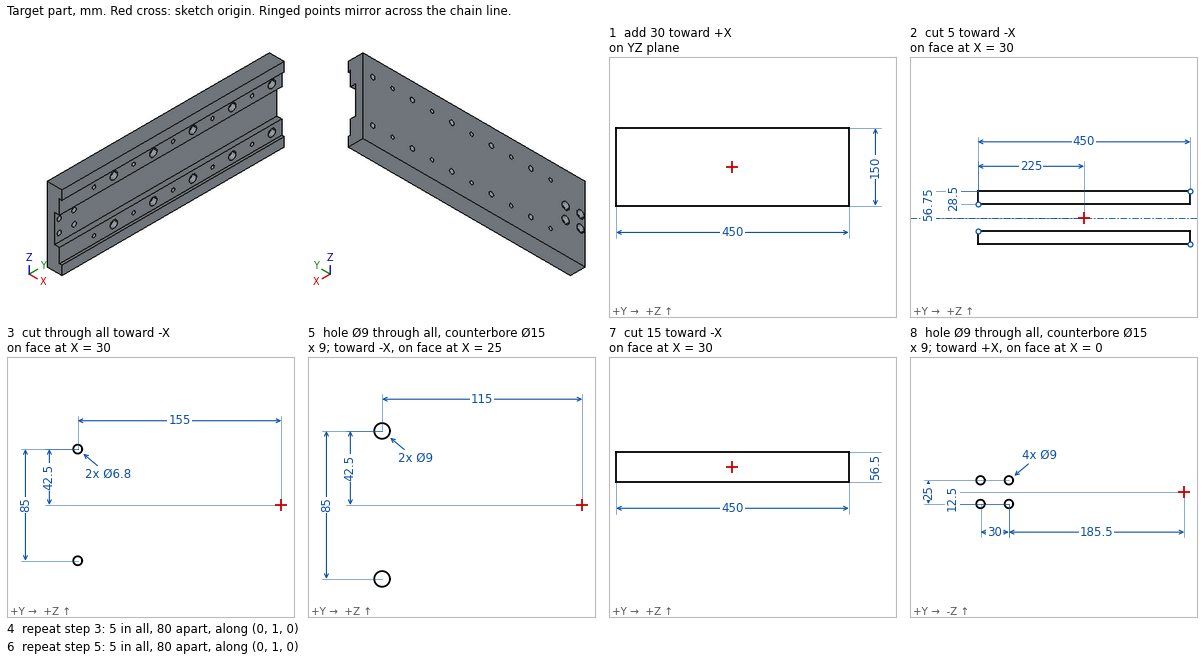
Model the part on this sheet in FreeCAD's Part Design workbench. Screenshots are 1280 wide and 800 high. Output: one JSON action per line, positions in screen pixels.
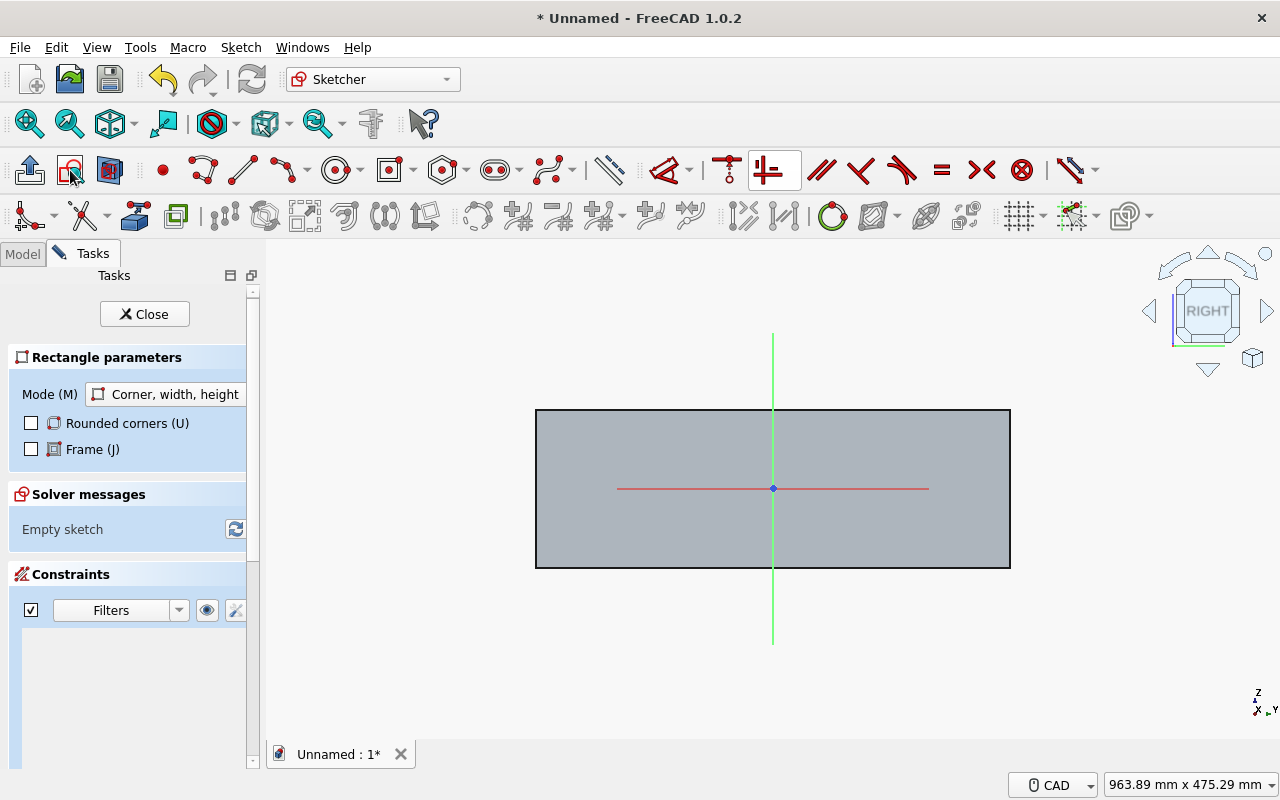
{"action": "left_click", "coordinate": [536, 429]}
{"action": "left_click", "coordinate": [1010, 459]}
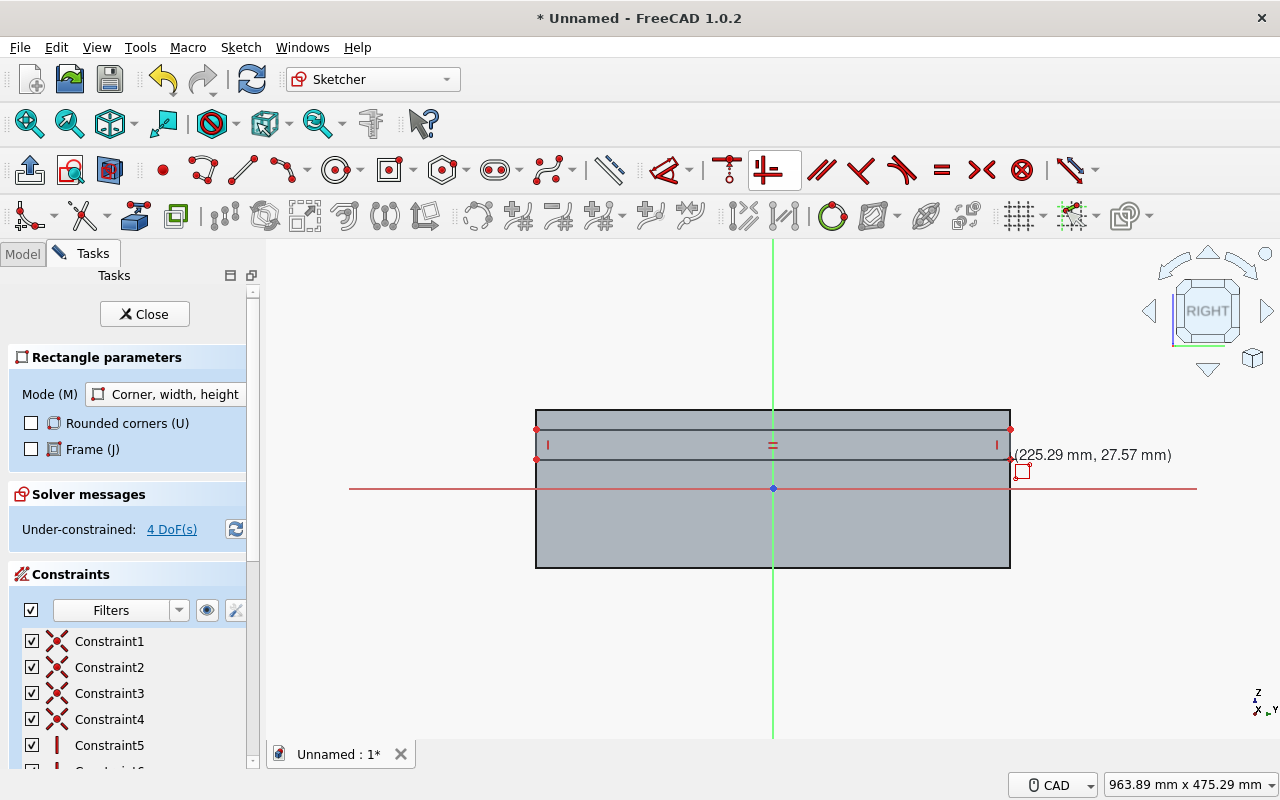
{"action": "left_click", "coordinate": [536, 519]}
{"action": "left_click", "coordinate": [1010, 549]}
{"action": "key", "text": "Escape"}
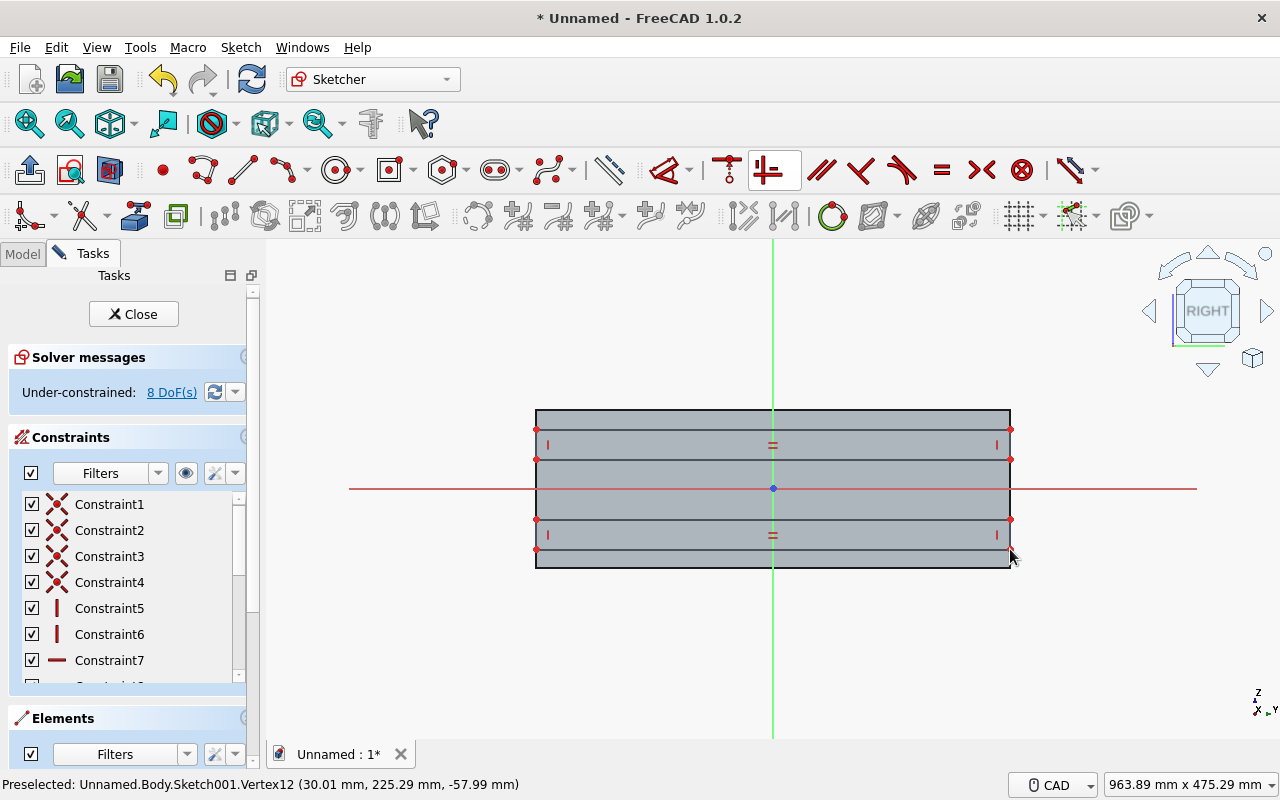
{"action": "left_click", "coordinate": [536, 460]}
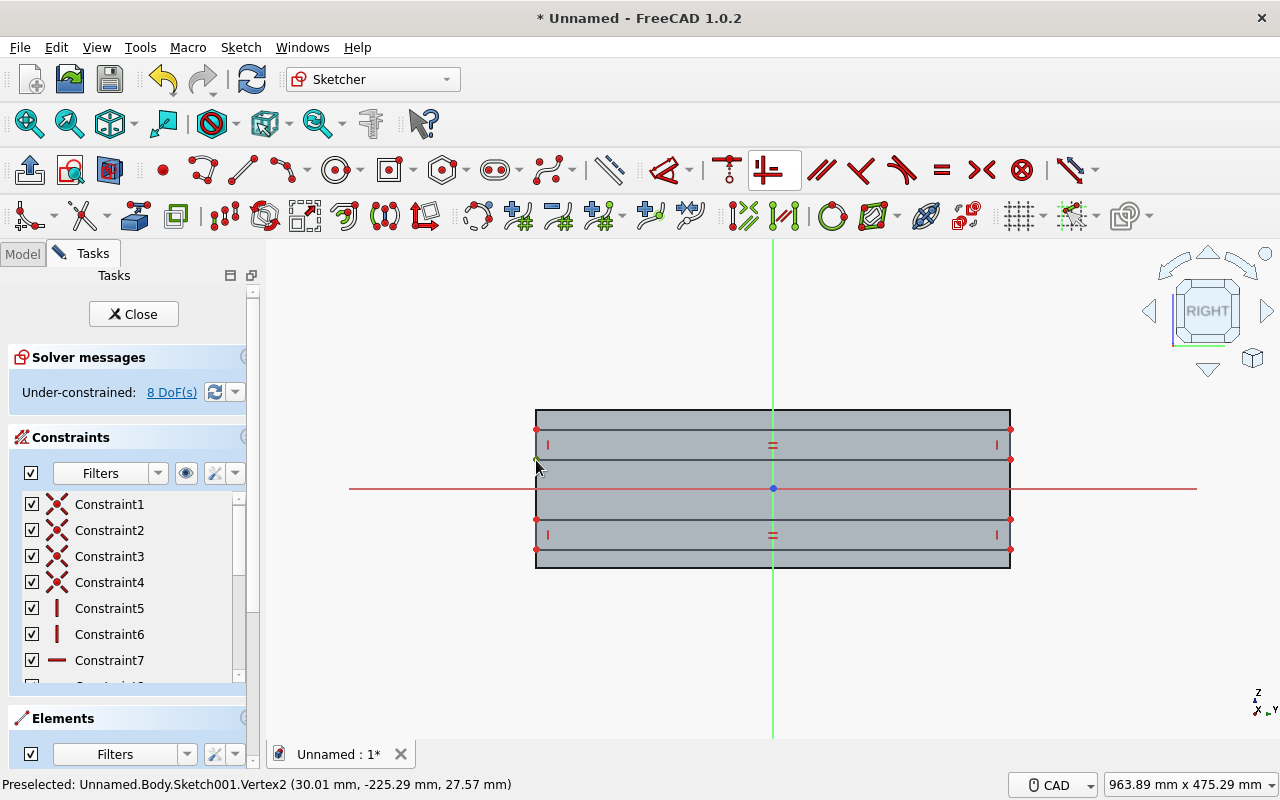
{"action": "left_click", "coordinate": [536, 520]}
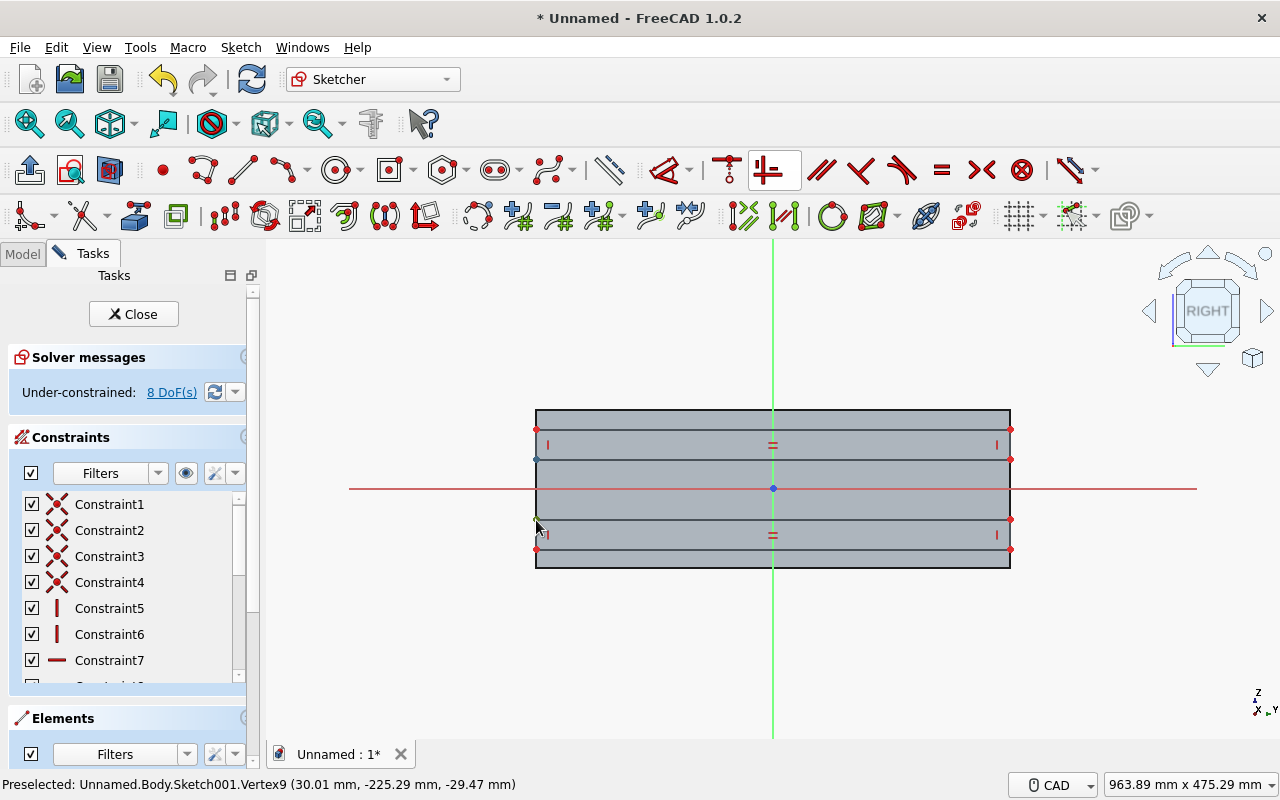
{"action": "left_click", "coordinate": [353, 489]}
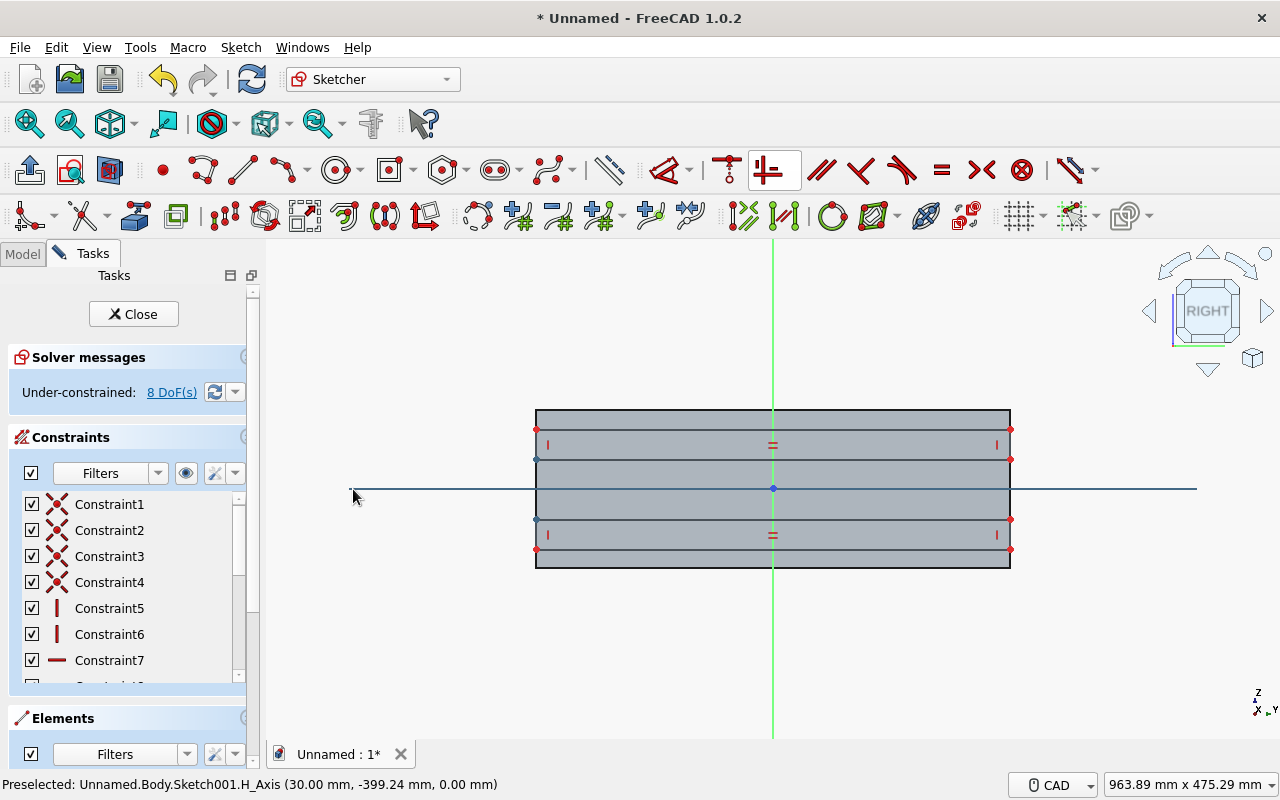
{"action": "left_click", "coordinate": [982, 170]}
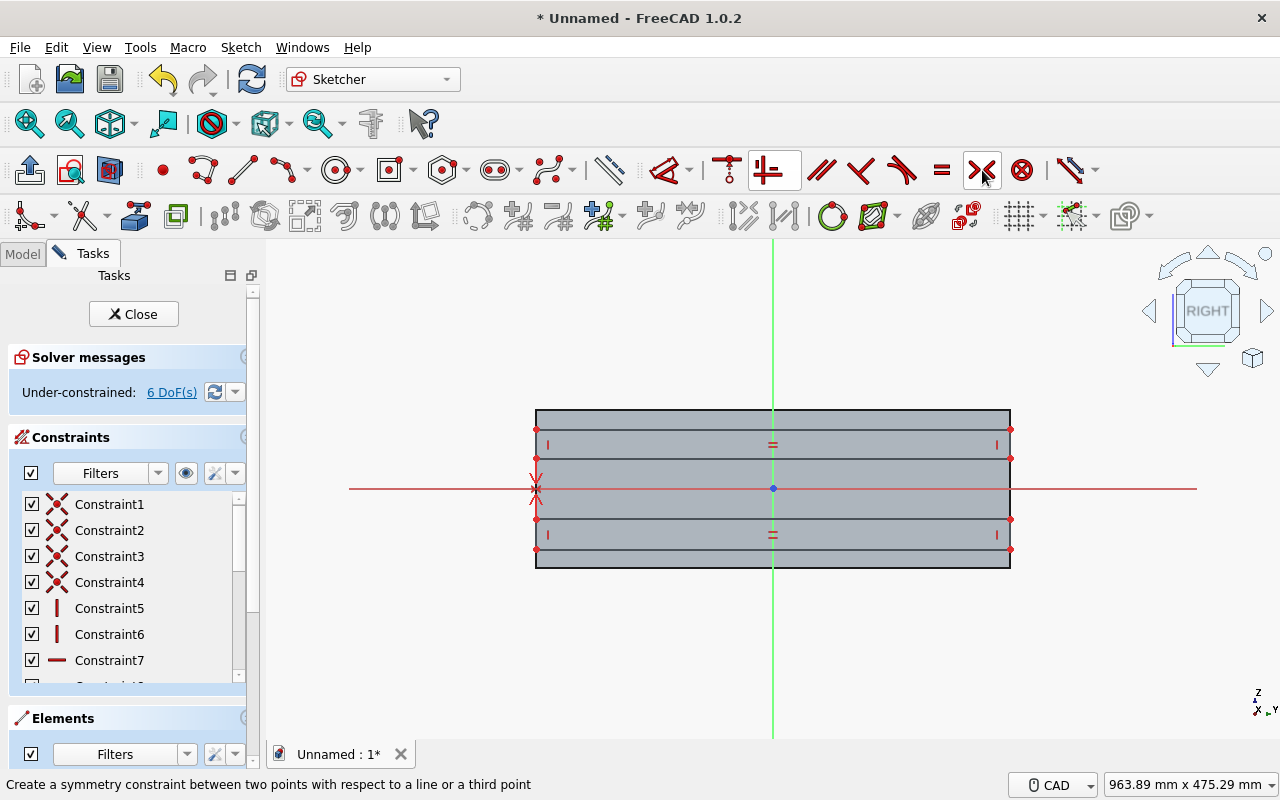
{"action": "left_click", "coordinate": [1010, 430]}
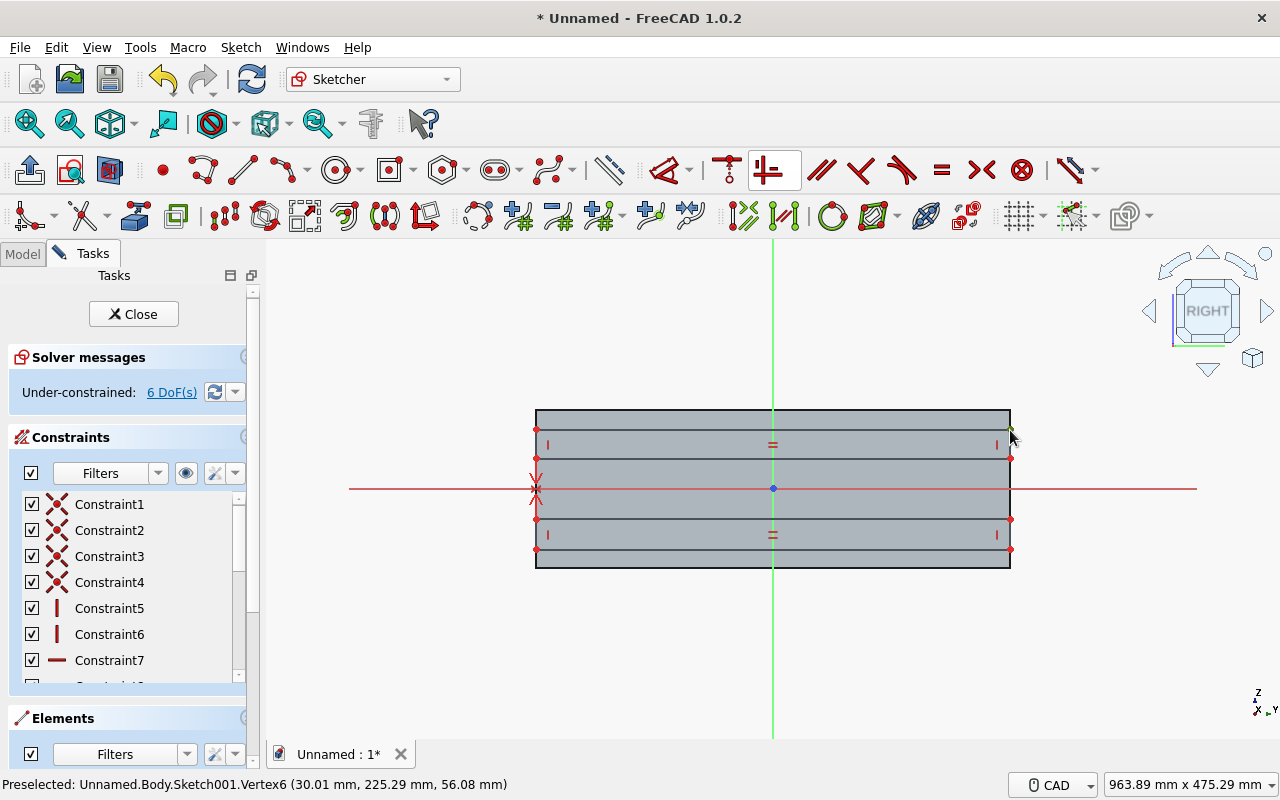
{"action": "left_click", "coordinate": [1010, 550]}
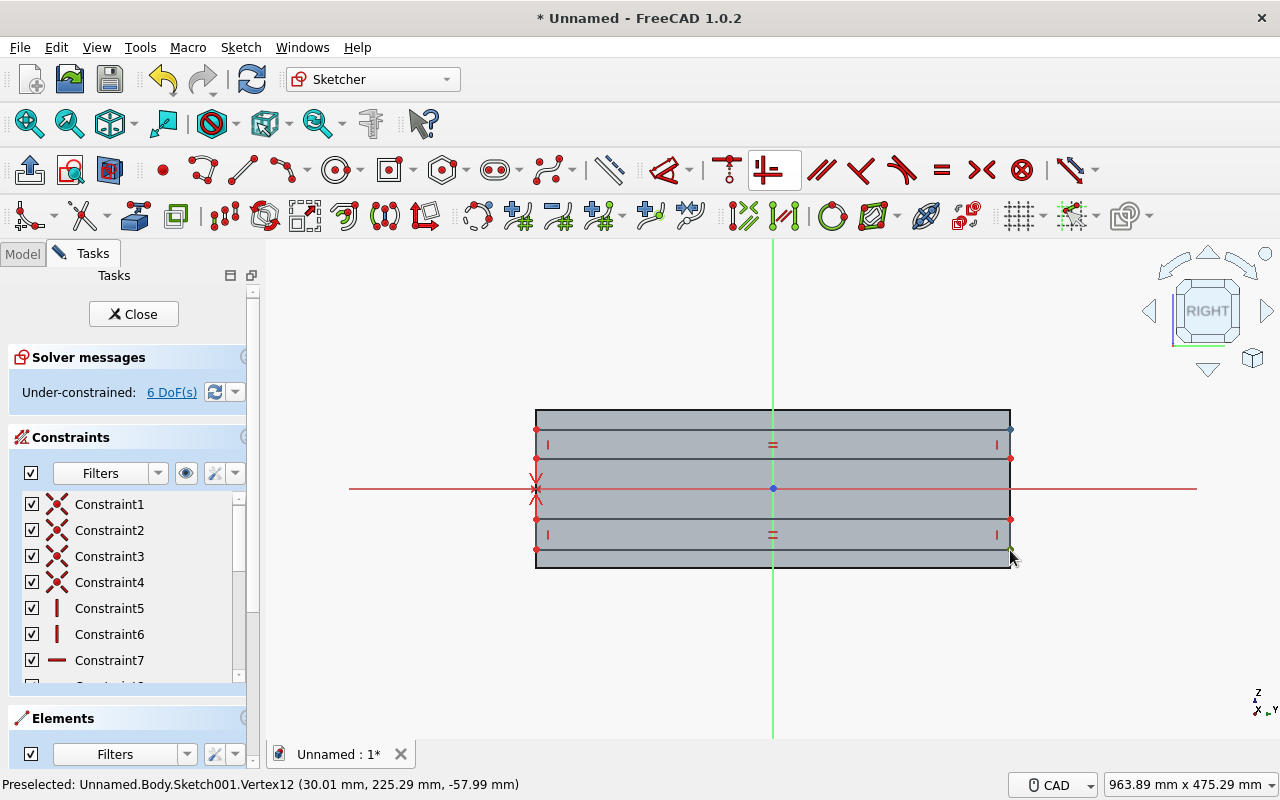
{"action": "left_click", "coordinate": [353, 489]}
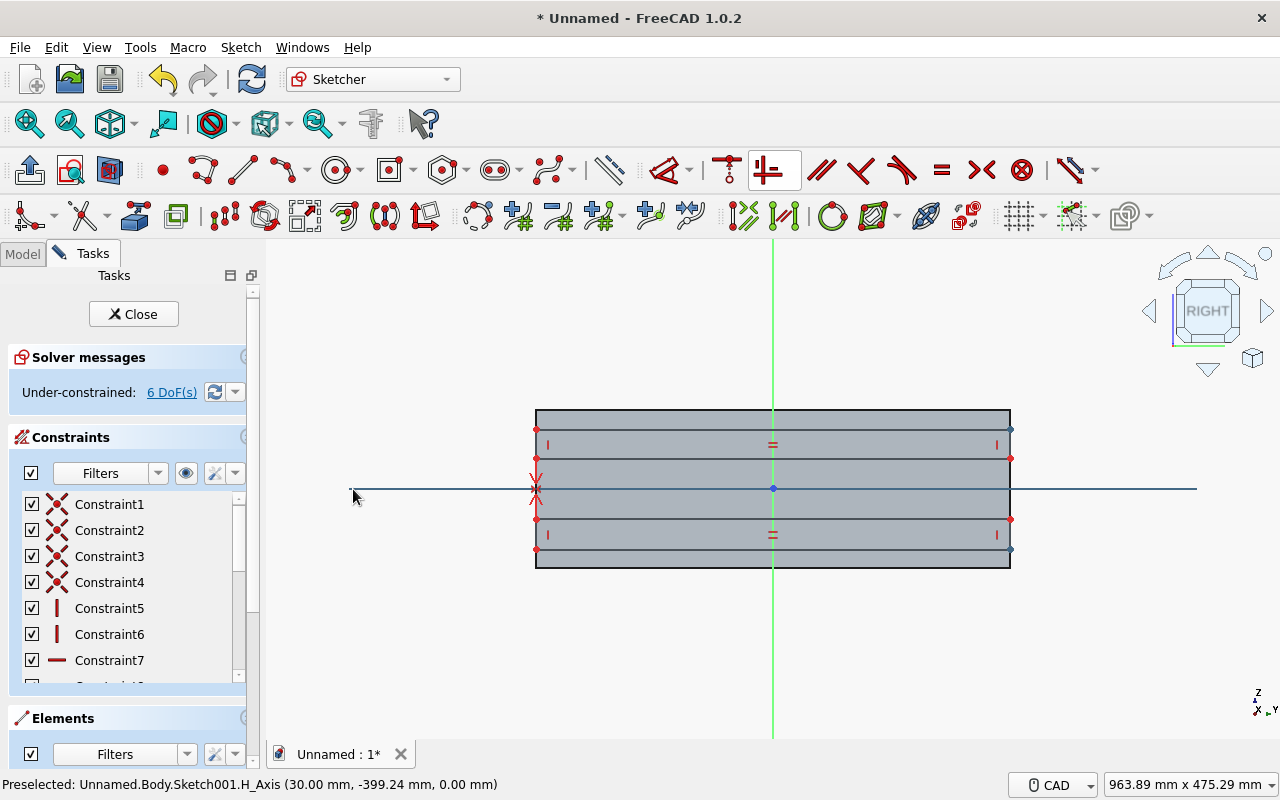
{"action": "left_click", "coordinate": [982, 170]}